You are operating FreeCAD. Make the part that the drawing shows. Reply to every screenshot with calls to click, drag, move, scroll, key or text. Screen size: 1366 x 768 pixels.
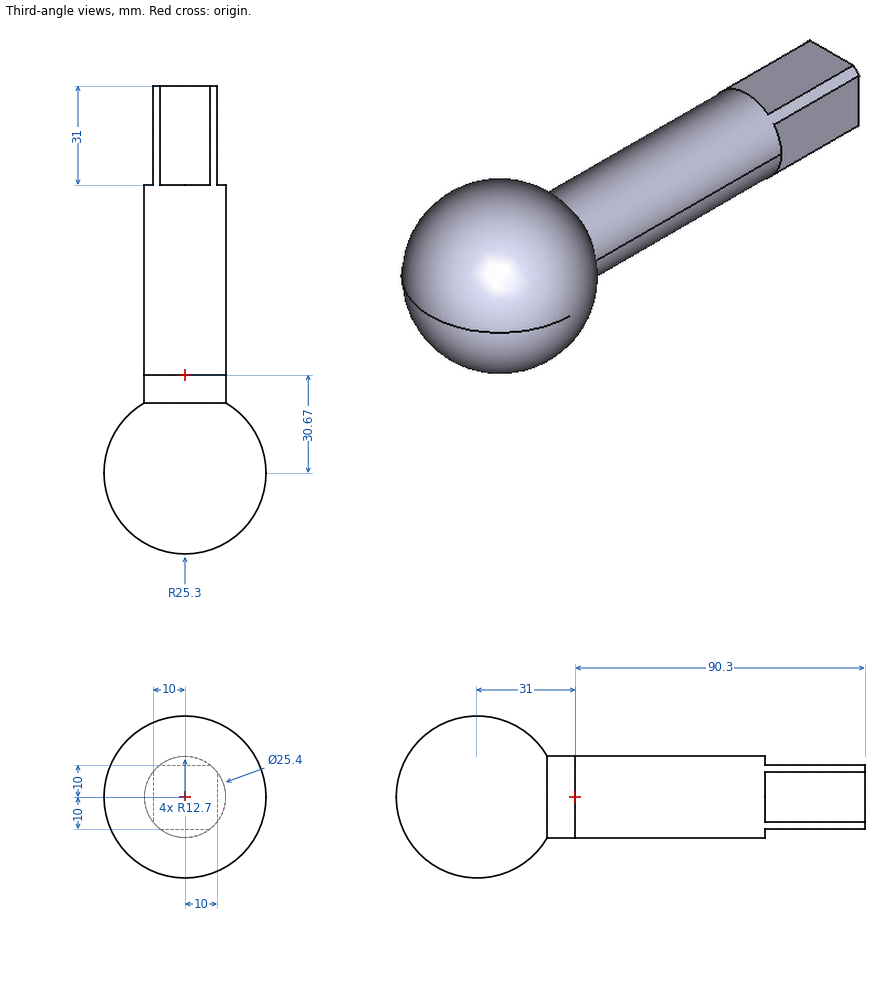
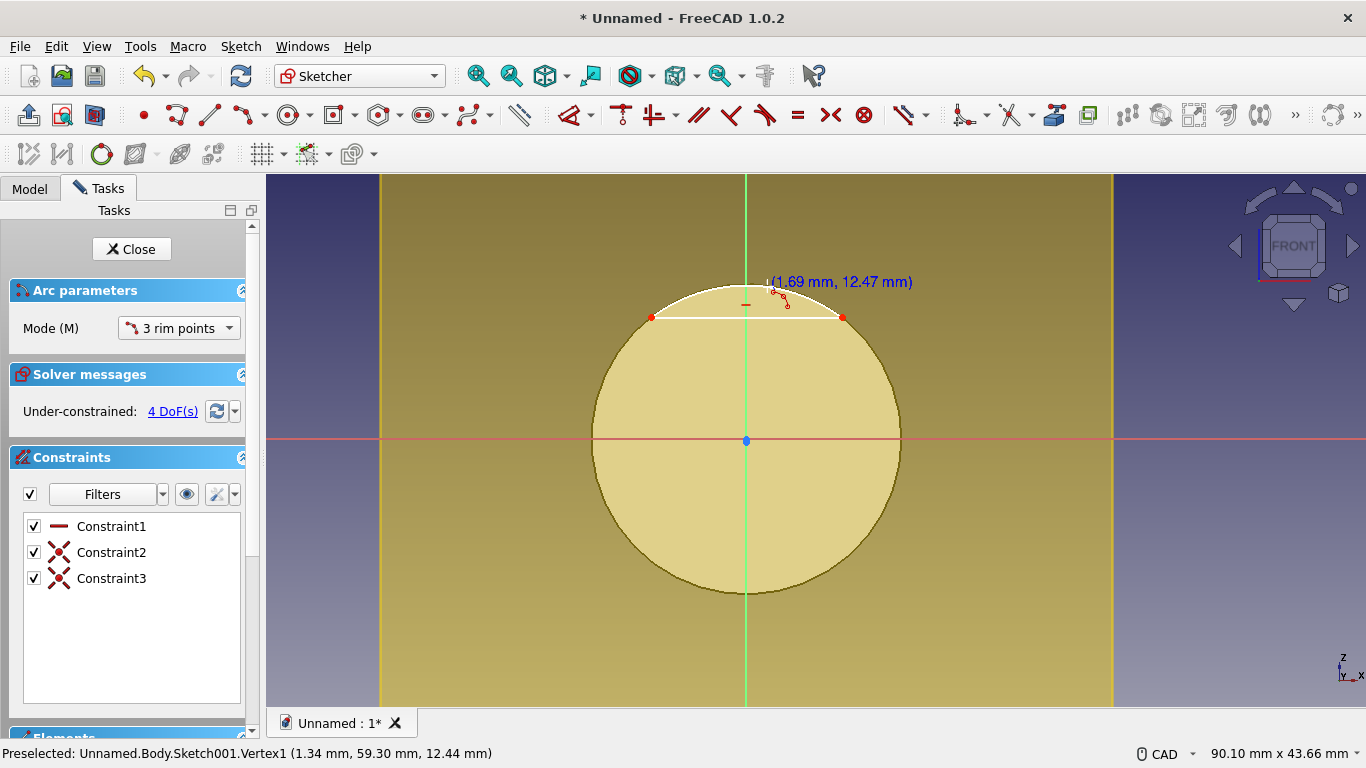
click(210, 116)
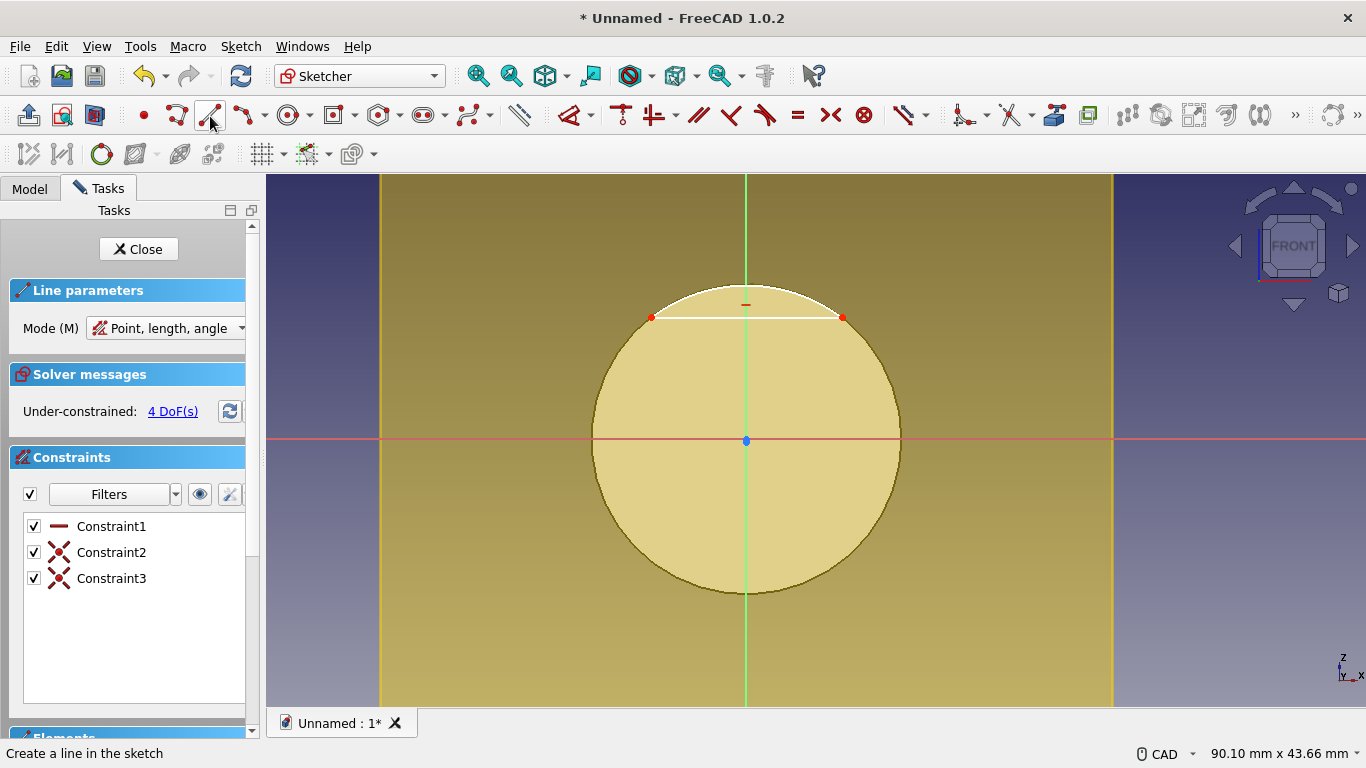
click(624, 344)
click(624, 535)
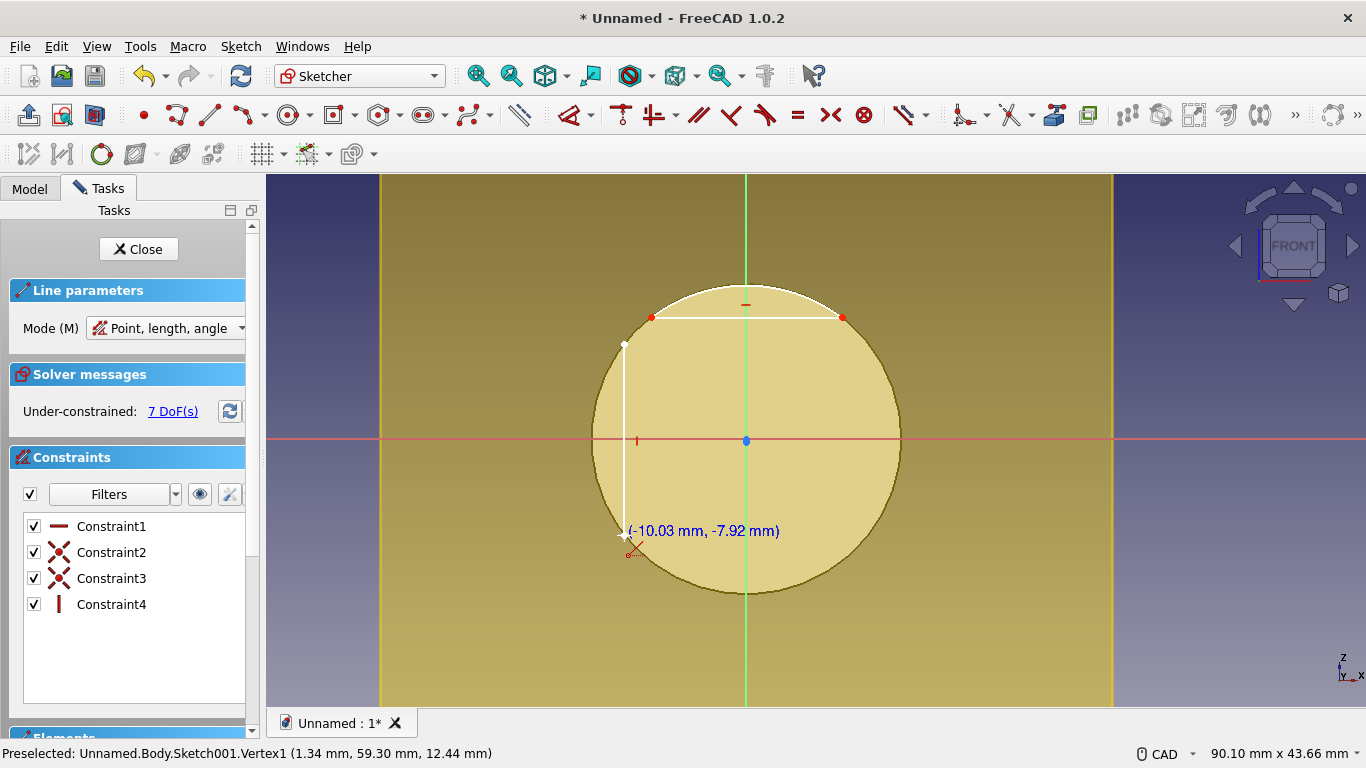
click(242, 116)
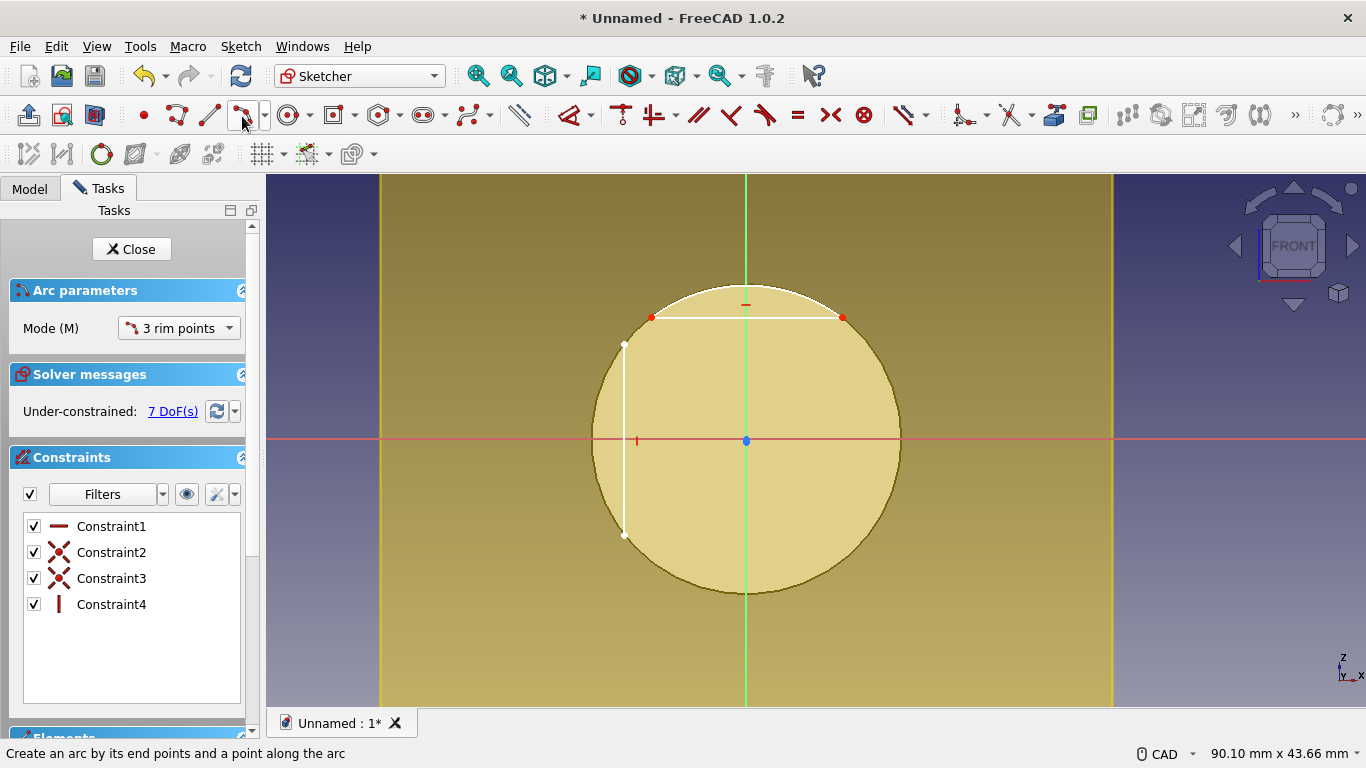
click(624, 536)
click(624, 345)
click(593, 419)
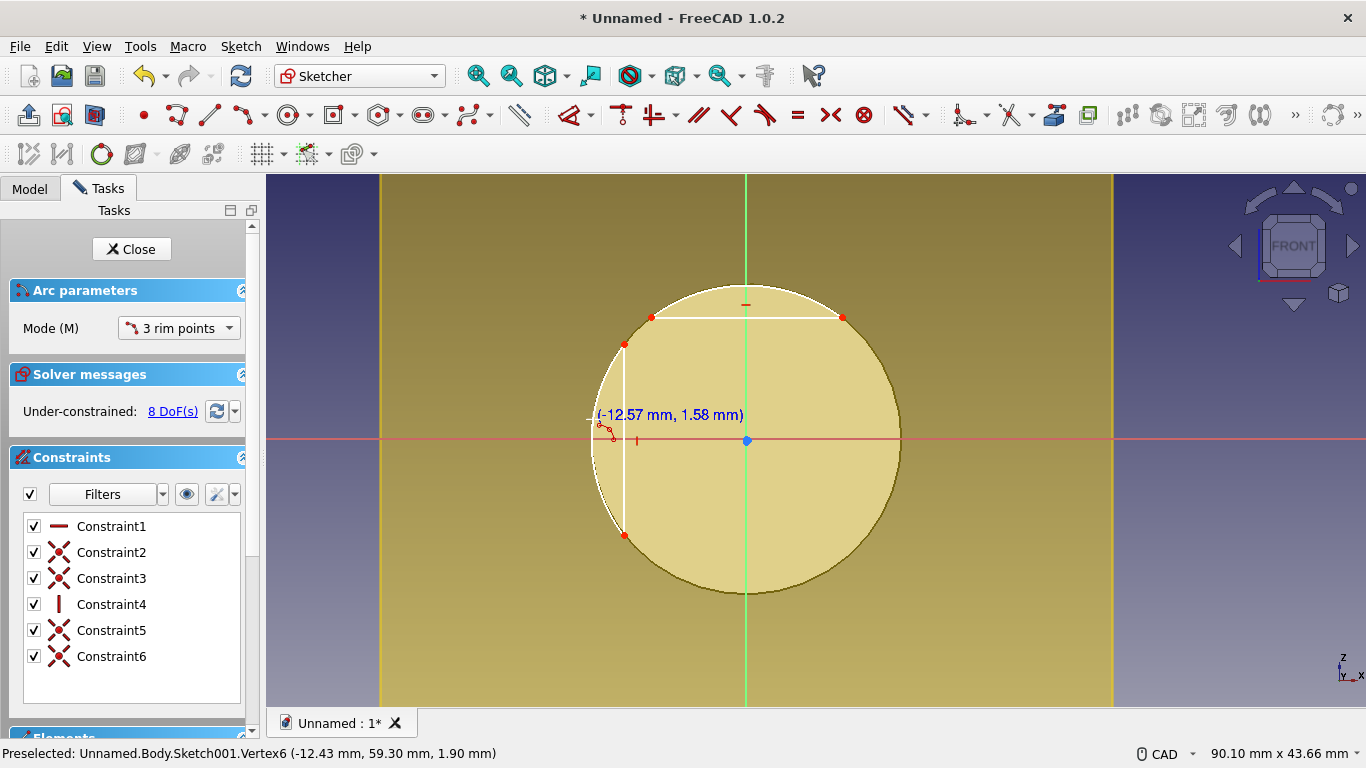
click(210, 116)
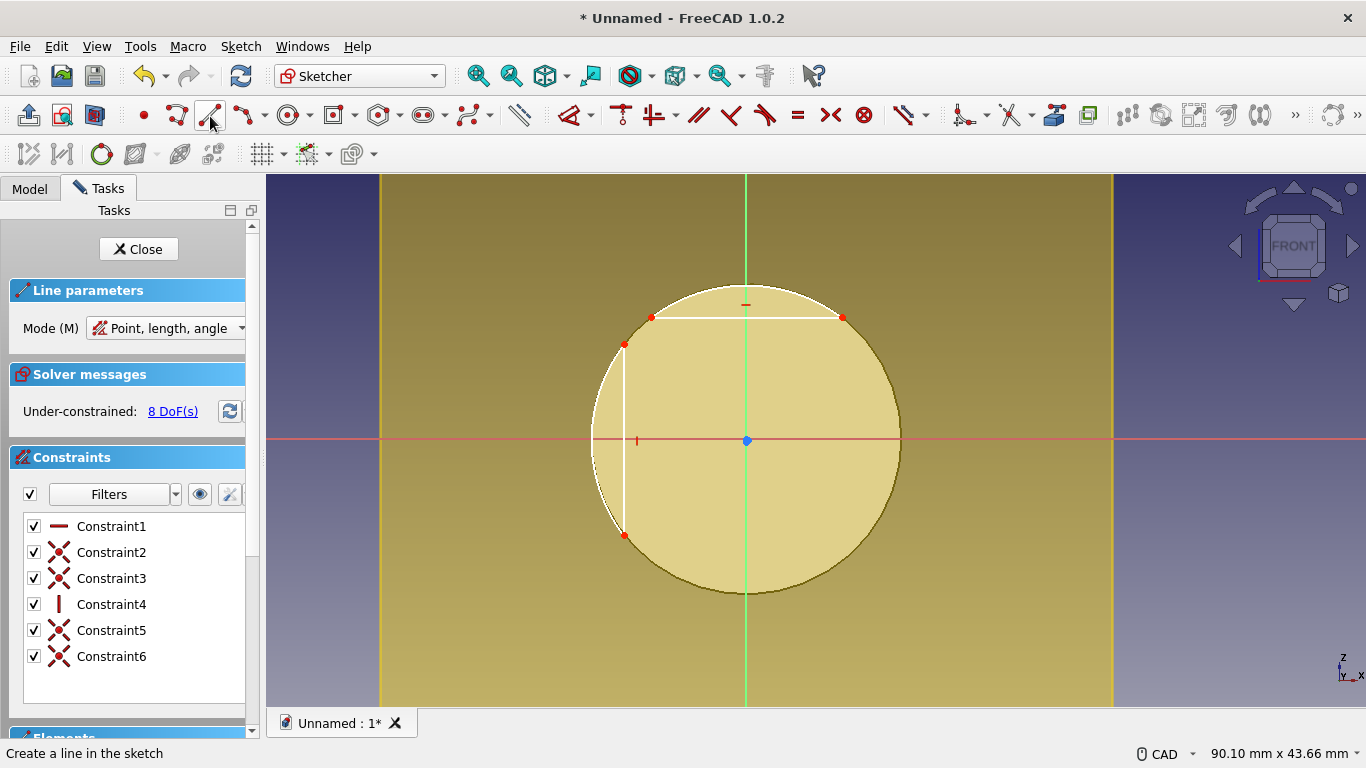
click(651, 561)
click(842, 561)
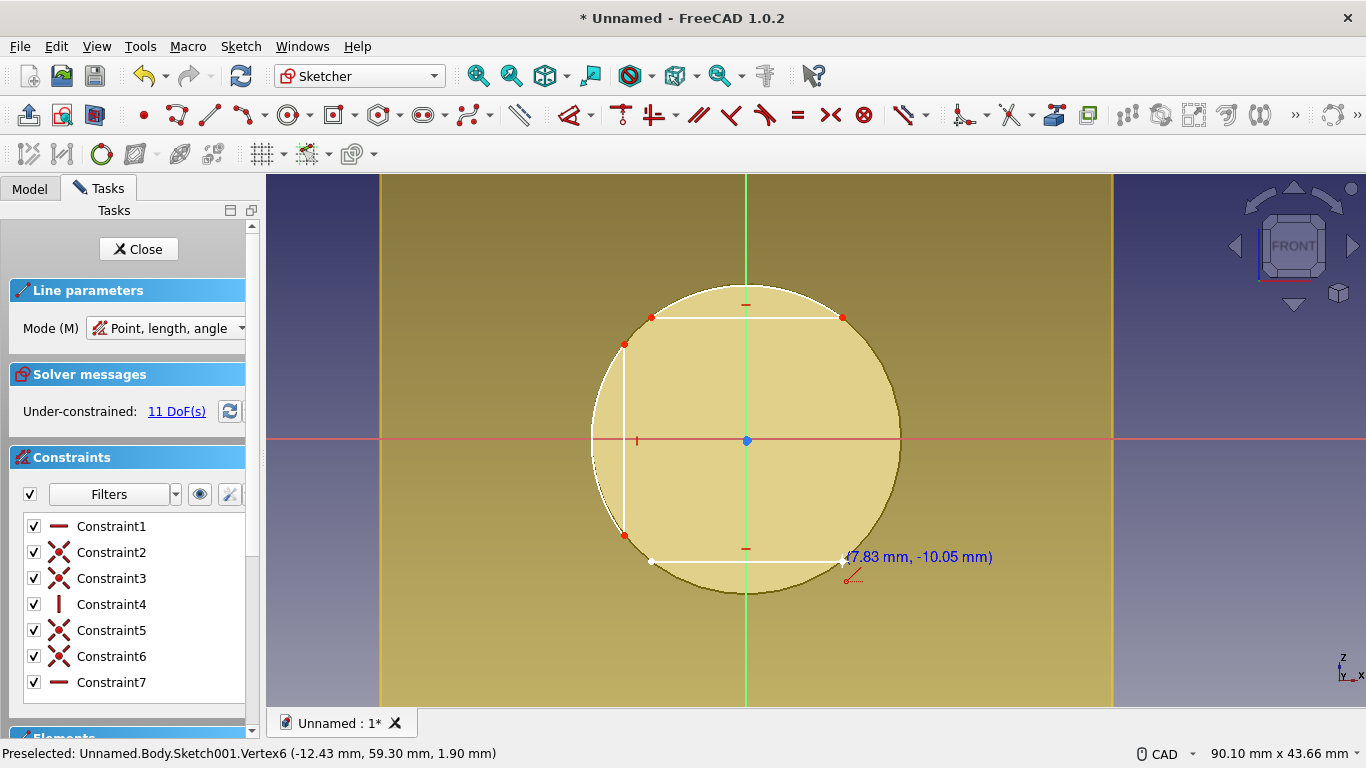
click(242, 116)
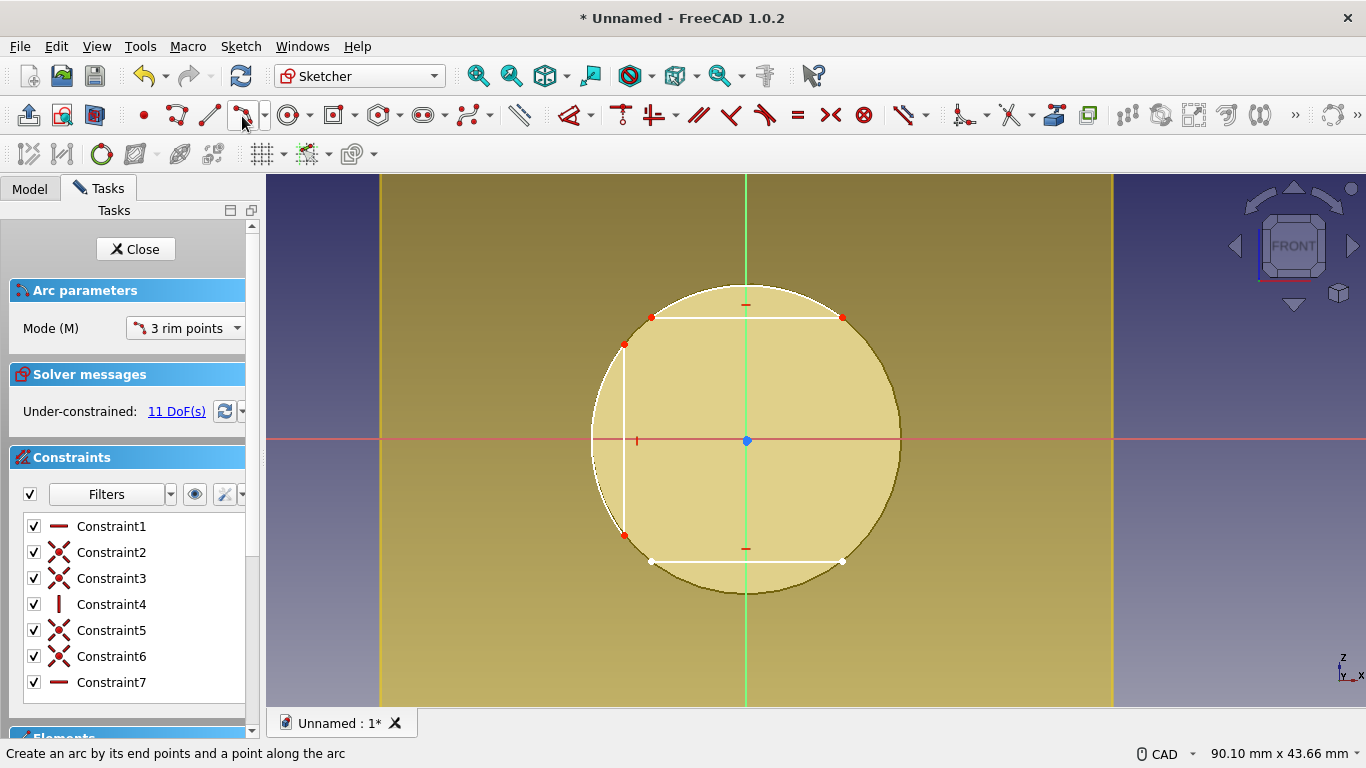
click(842, 562)
click(651, 562)
click(726, 593)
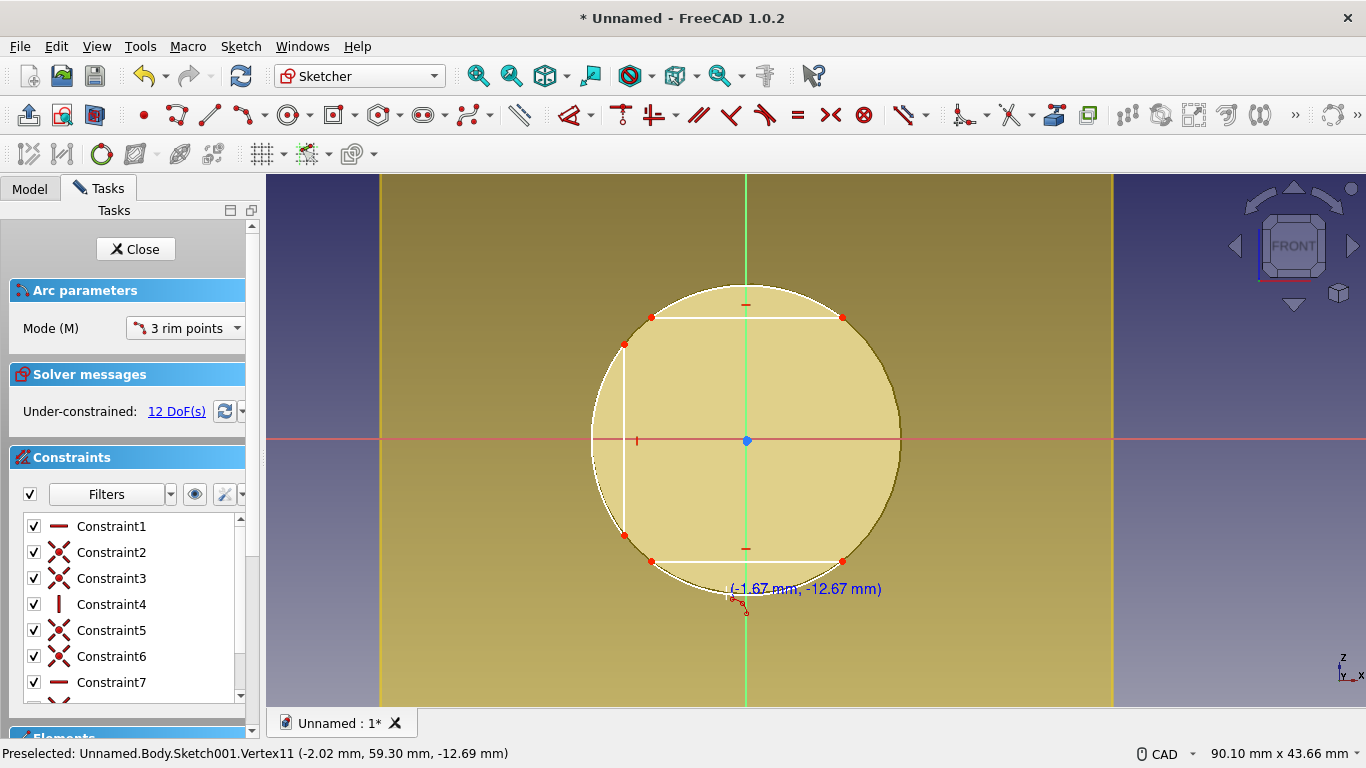
key(g)
key(l)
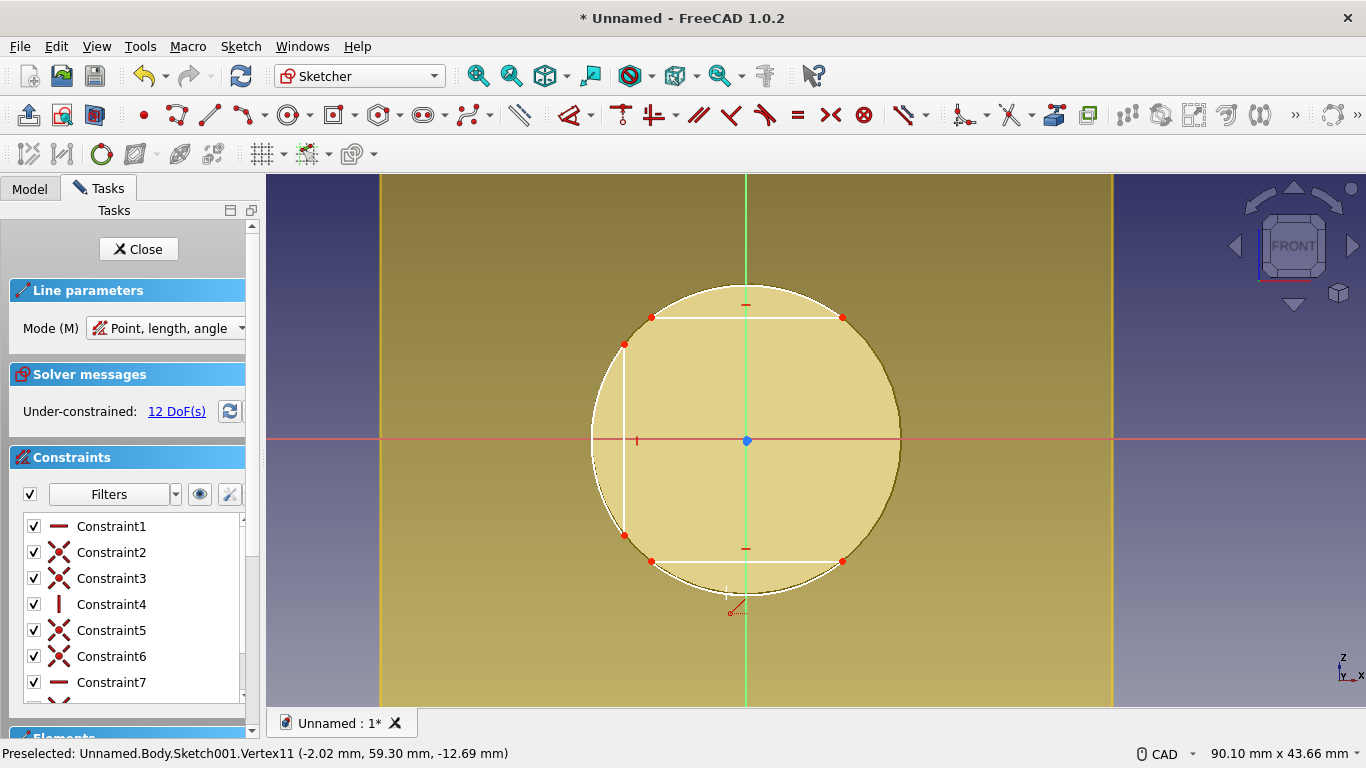
click(868, 535)
click(868, 344)